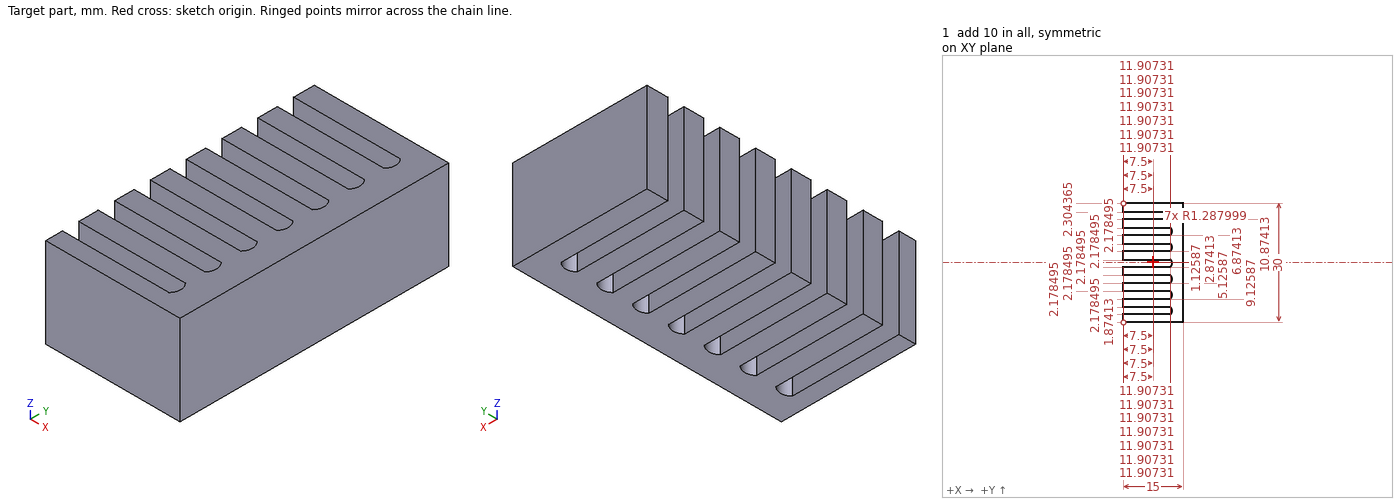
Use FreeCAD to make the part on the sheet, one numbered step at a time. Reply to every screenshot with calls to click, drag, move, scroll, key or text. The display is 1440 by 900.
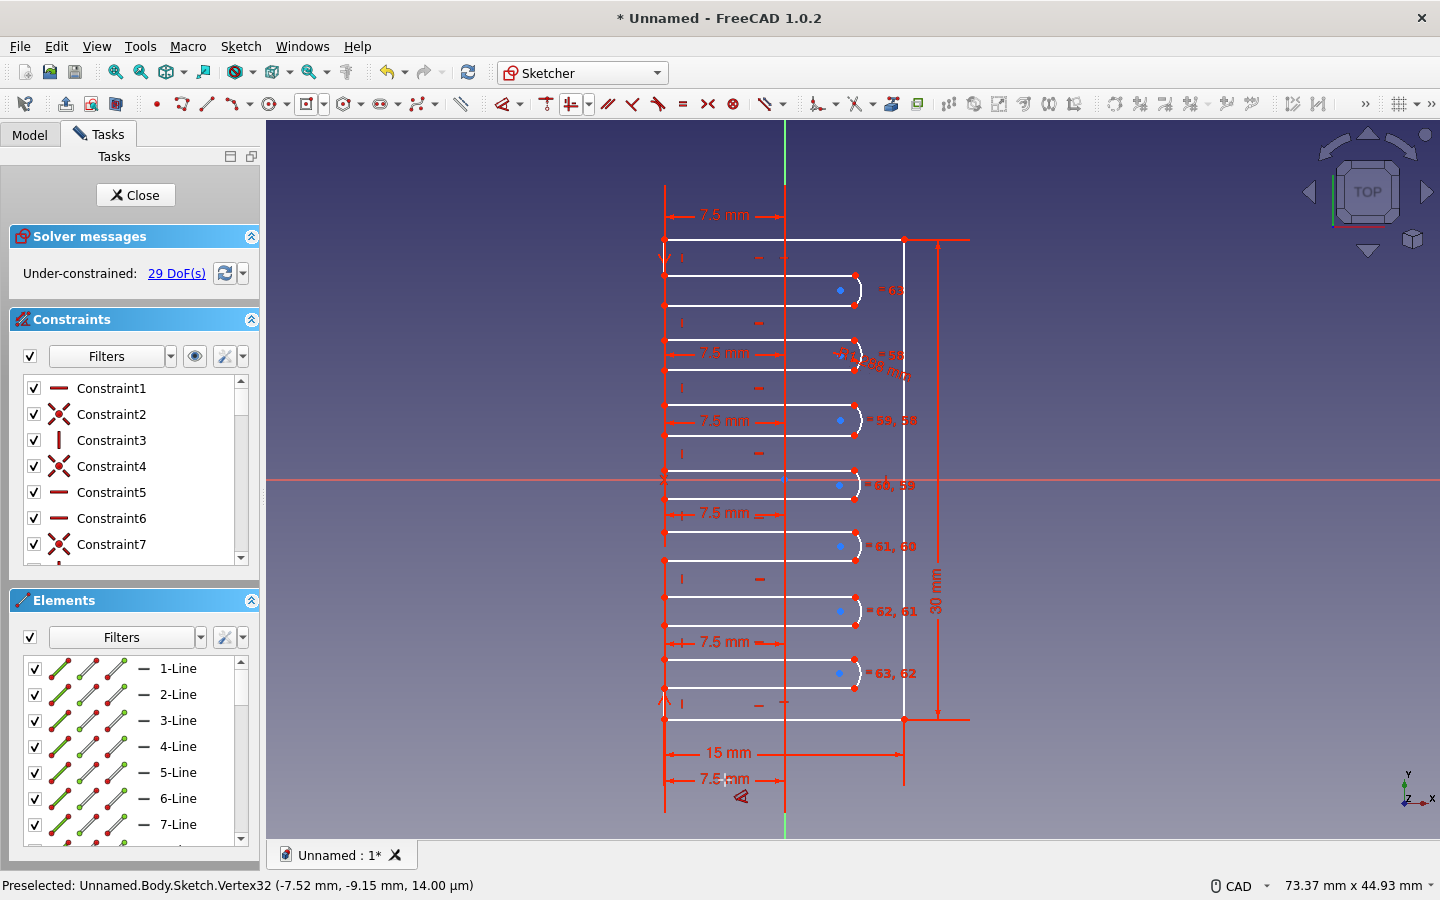
click(664, 688)
click(725, 326)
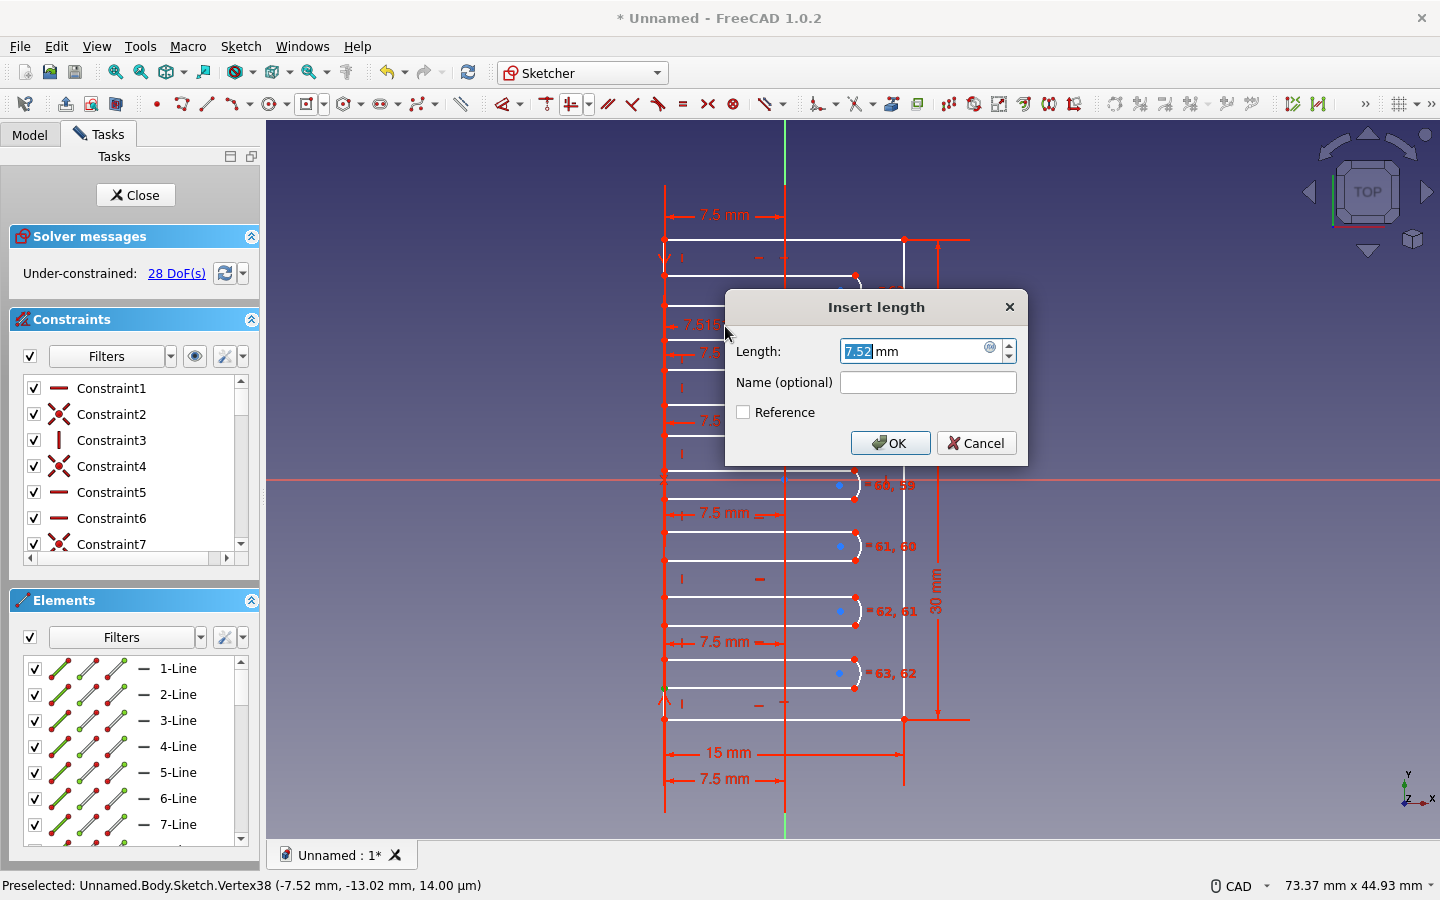
text(7.5)
key(Return)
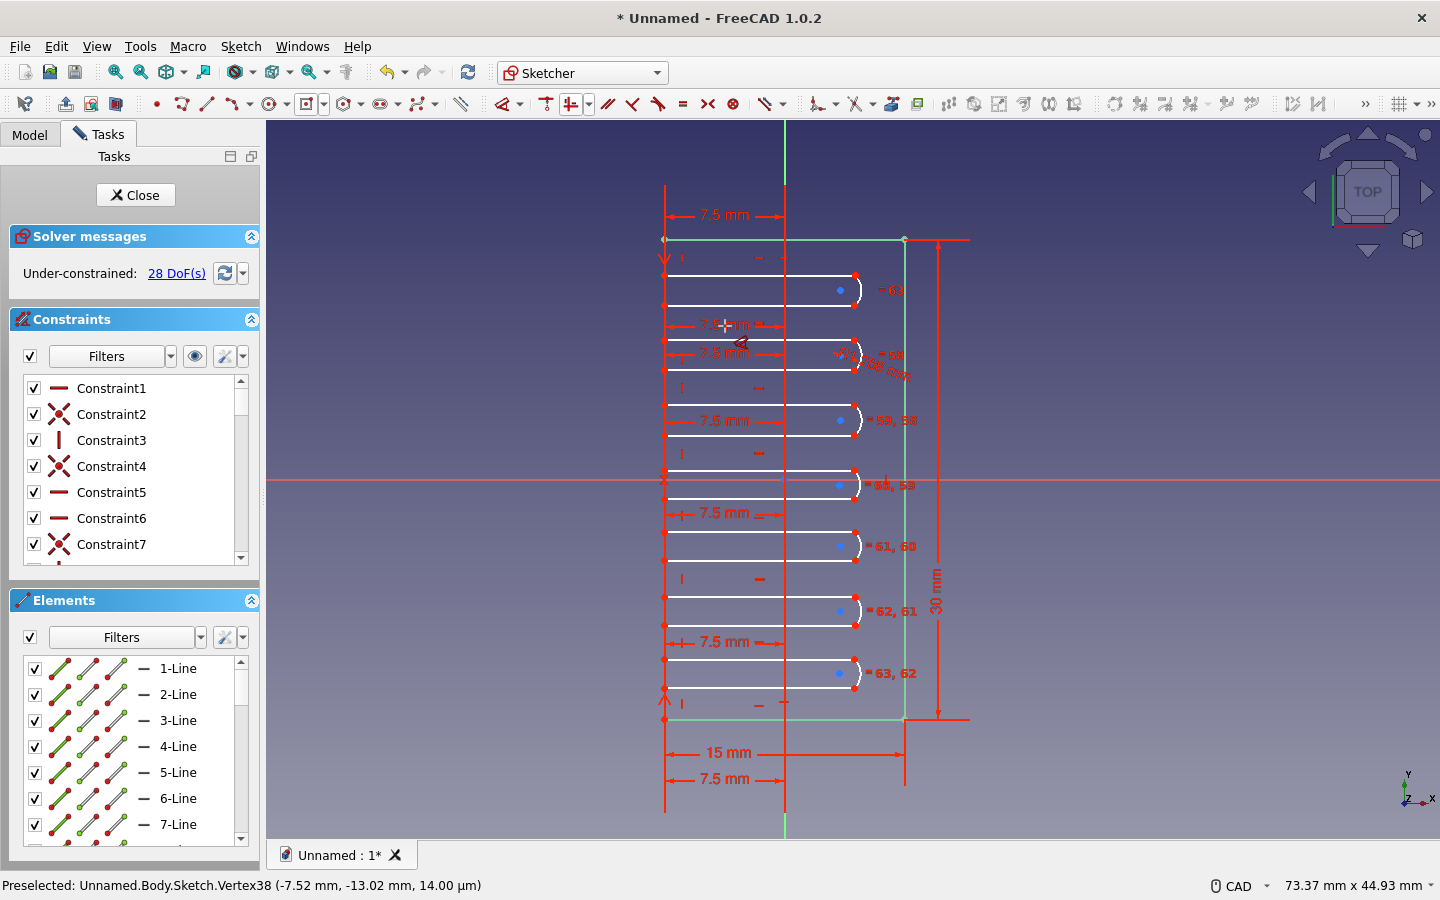
scroll(665, 697, up, 2)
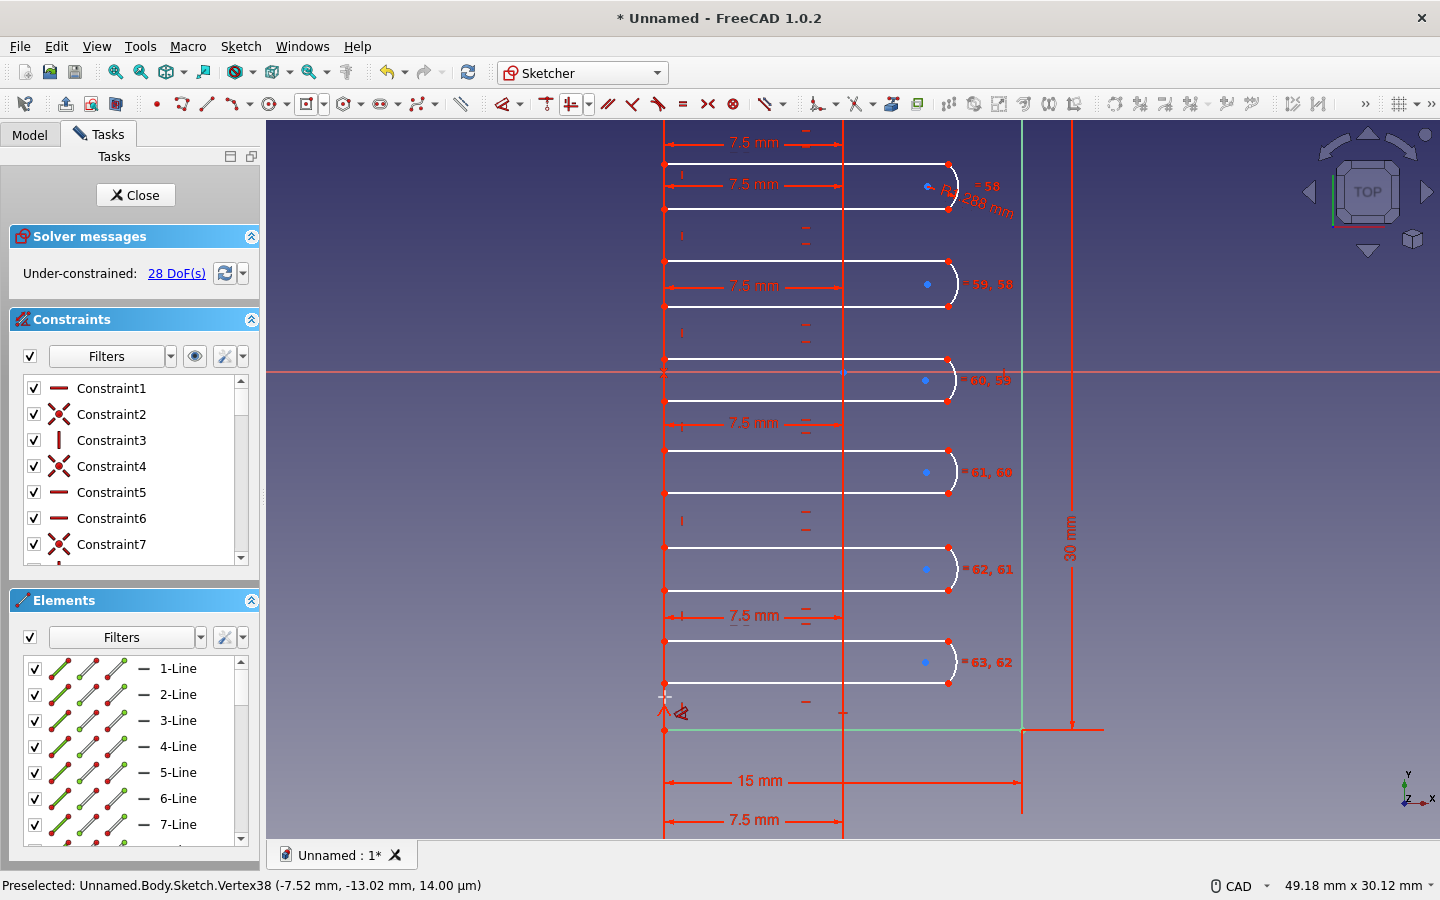
click(664, 697)
click(630, 707)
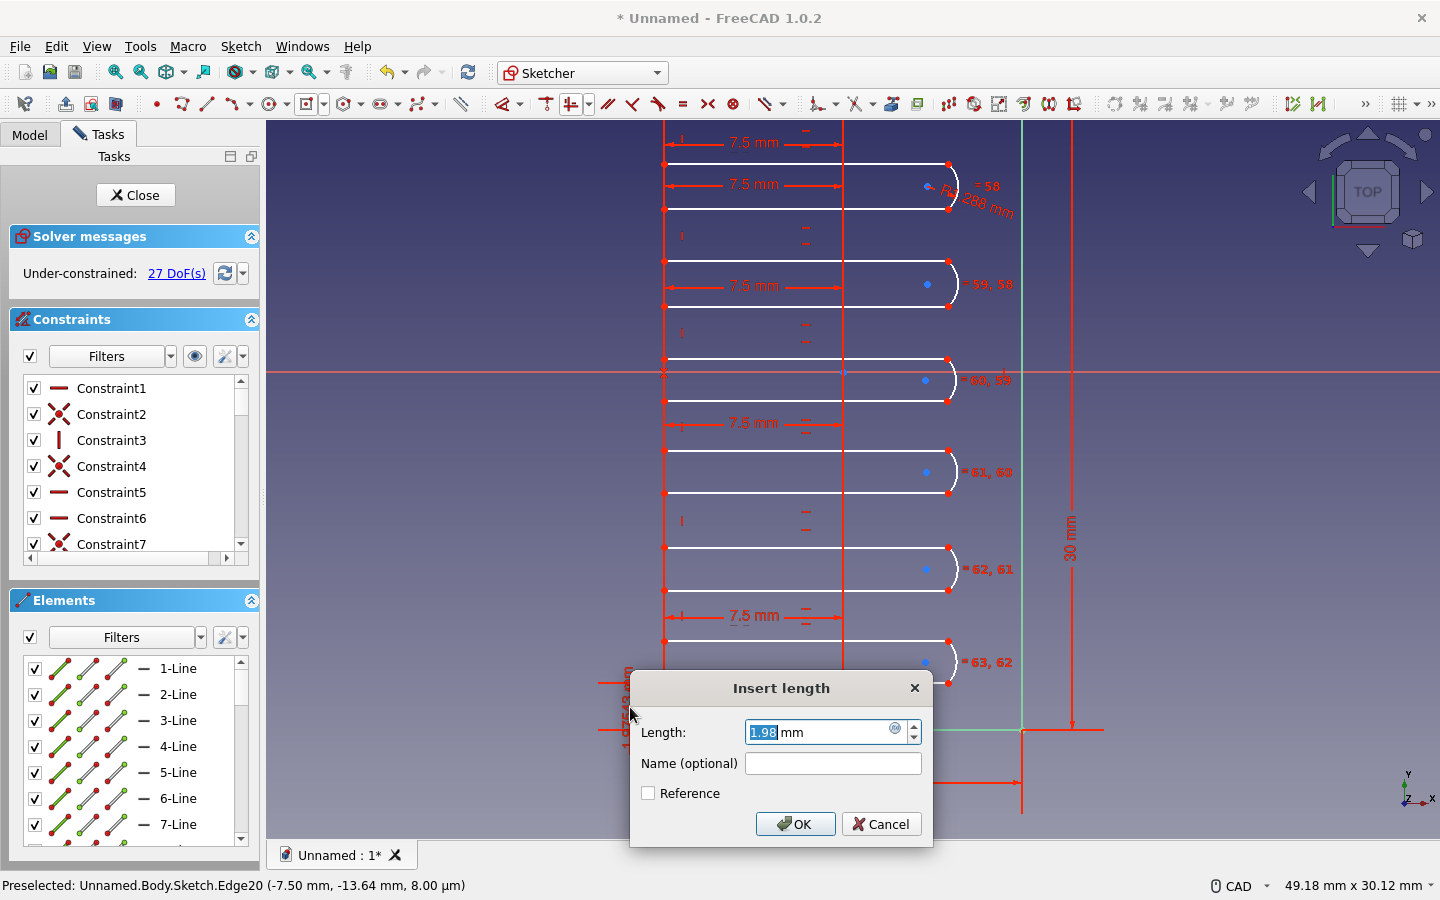
text(1.87413)
key(Return)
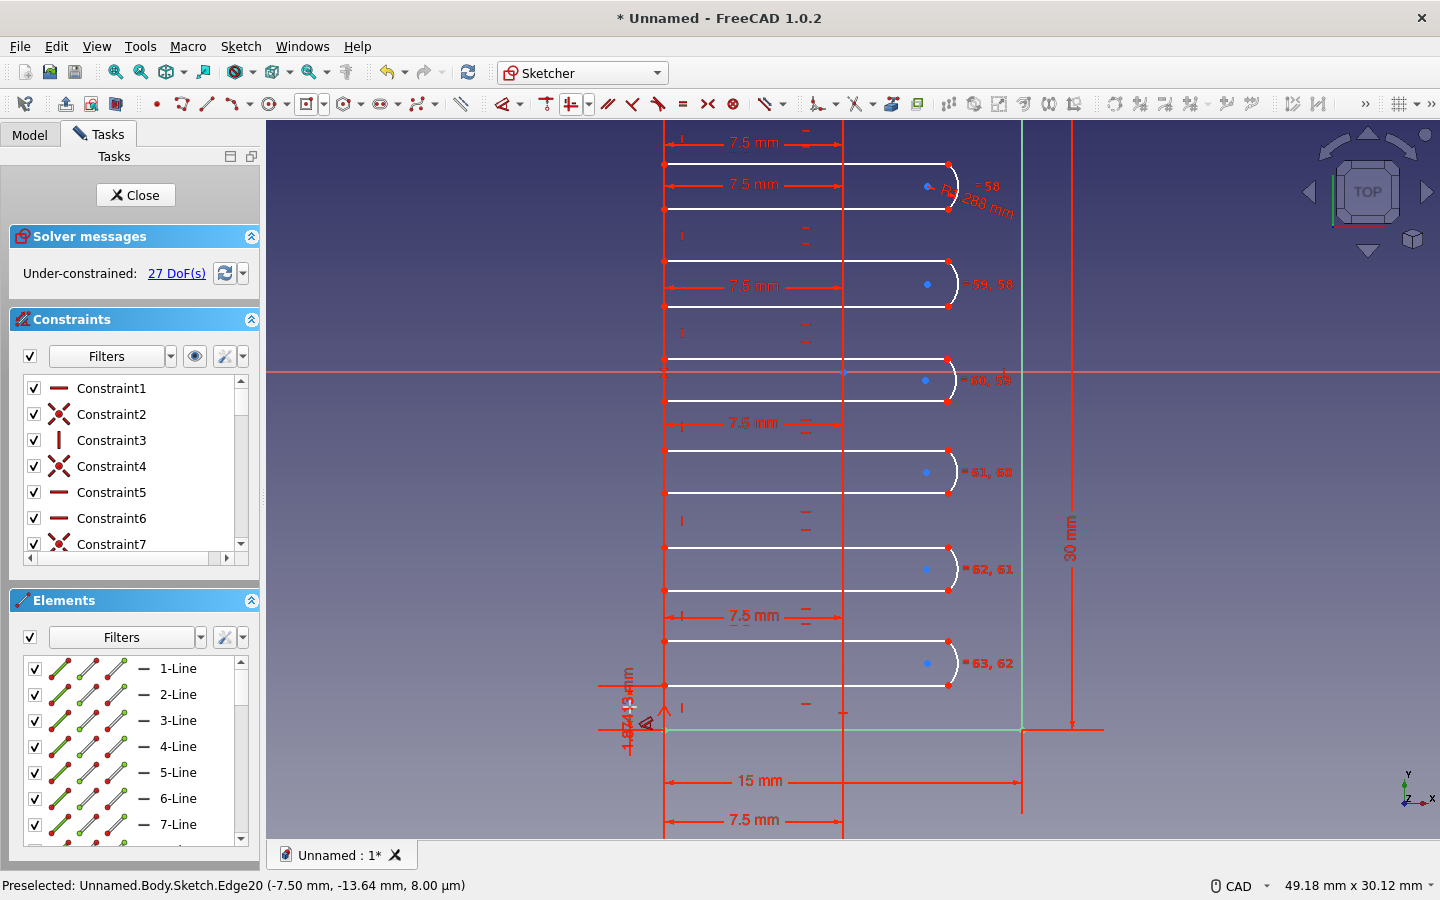
scroll(665, 698, down, 2)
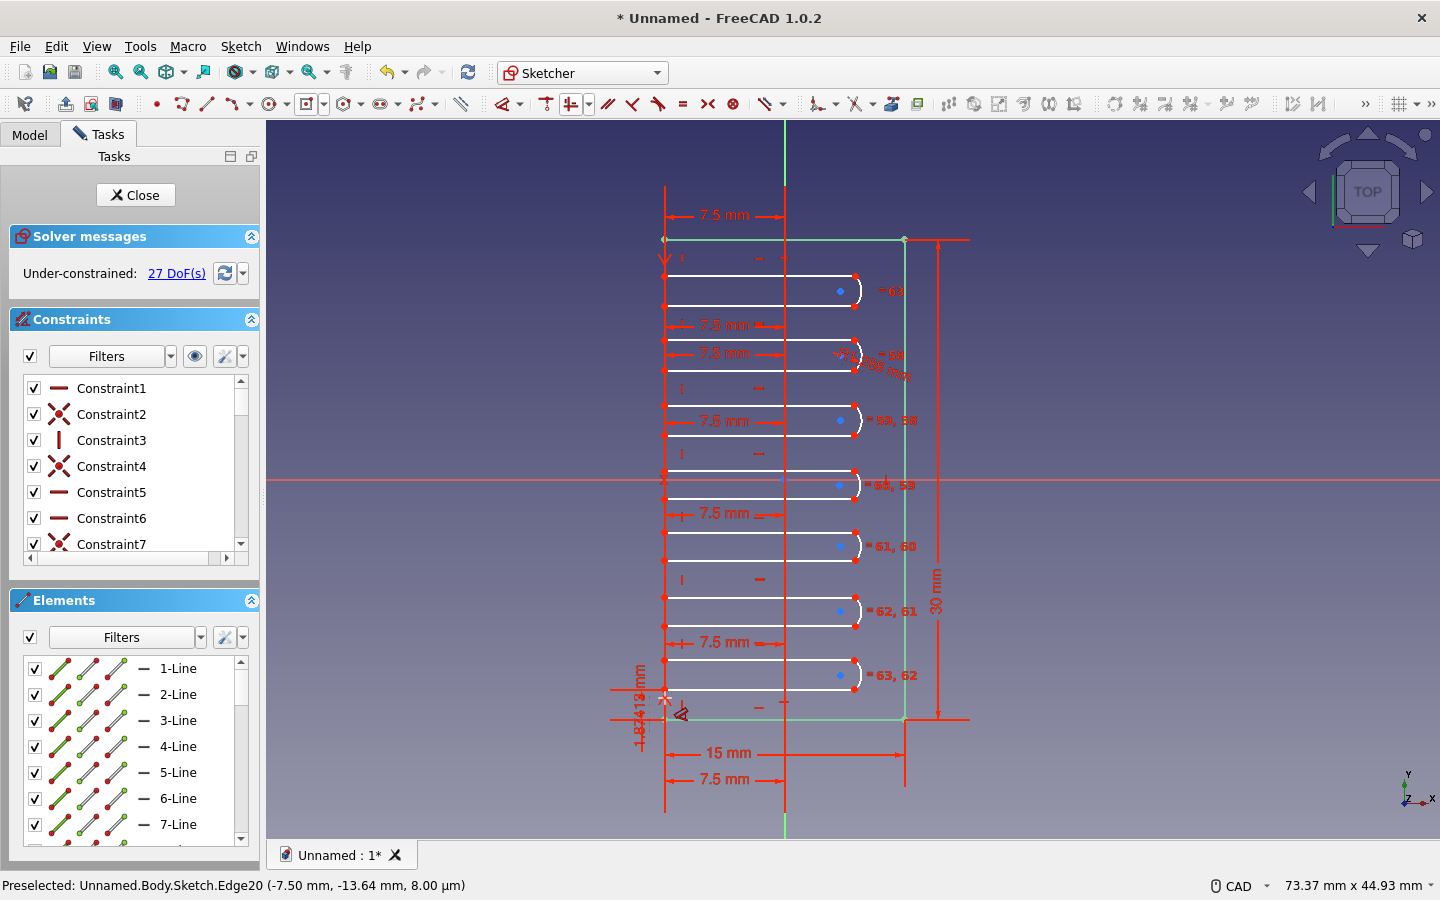
click(798, 306)
click(804, 224)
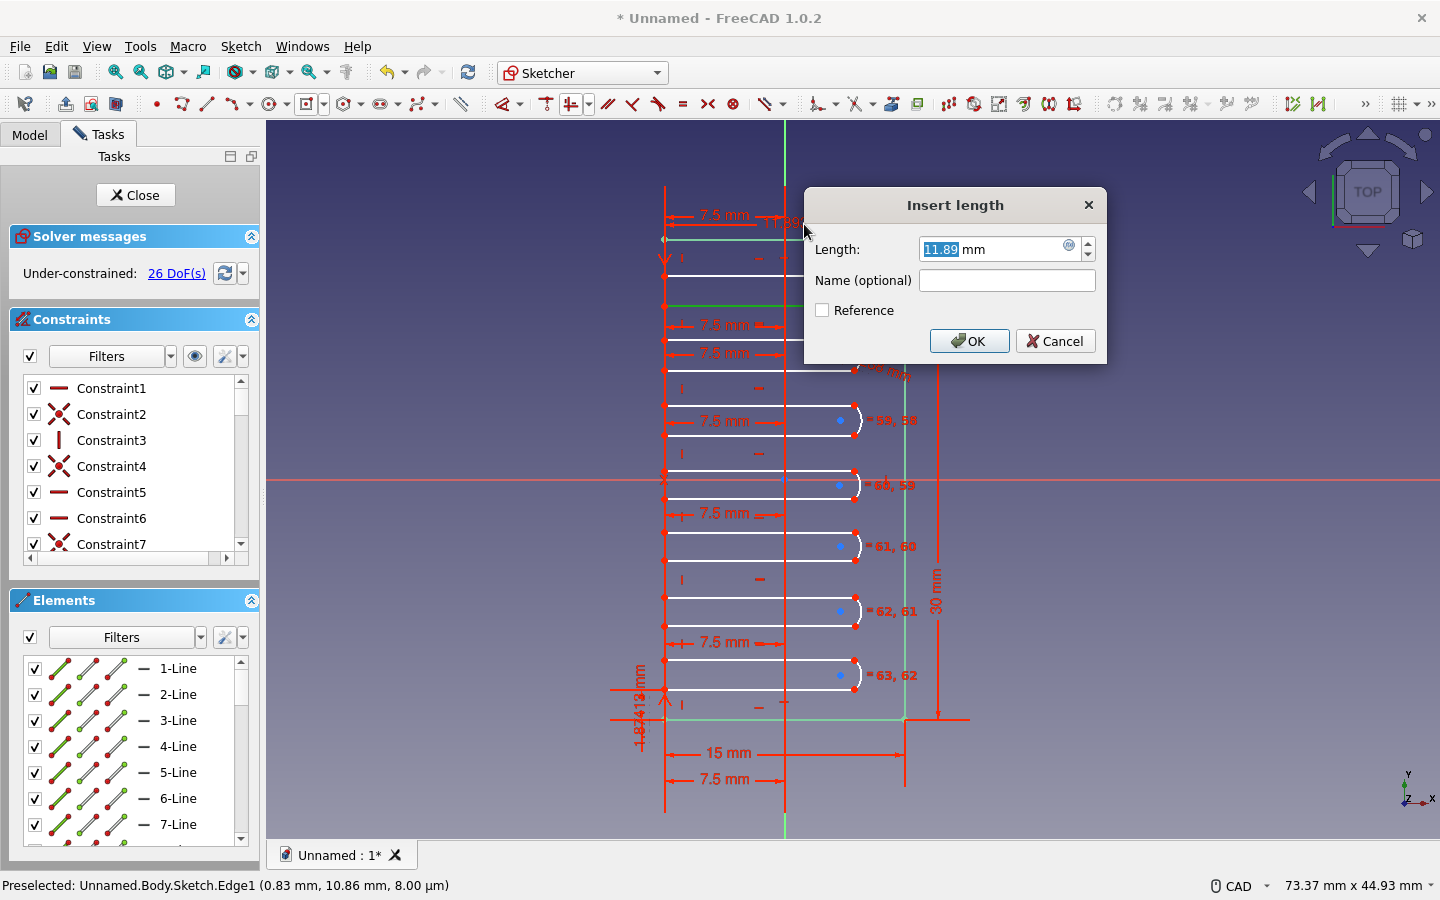
text(11.90731)
key(Return)